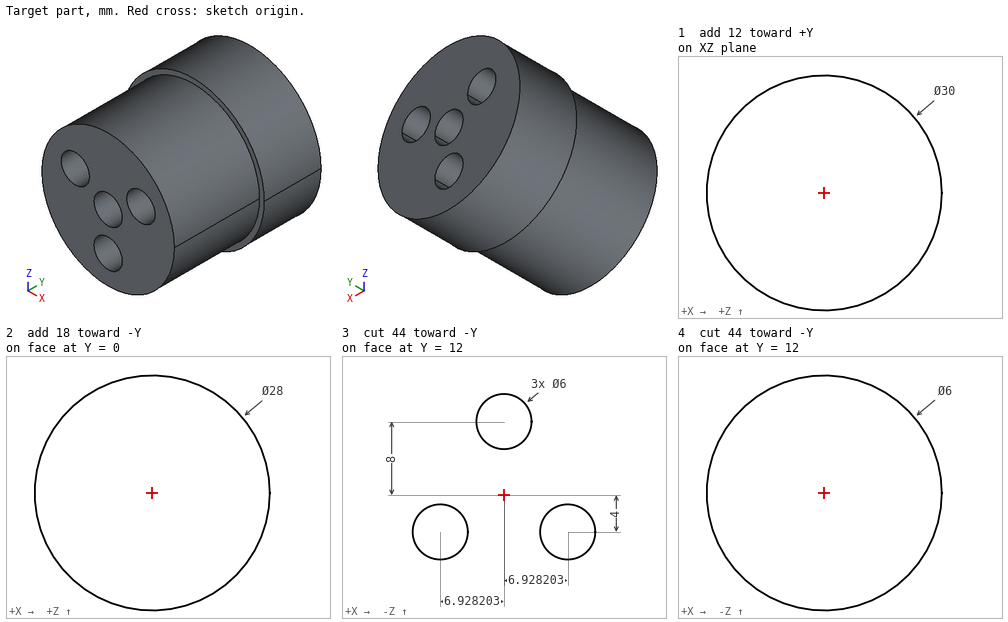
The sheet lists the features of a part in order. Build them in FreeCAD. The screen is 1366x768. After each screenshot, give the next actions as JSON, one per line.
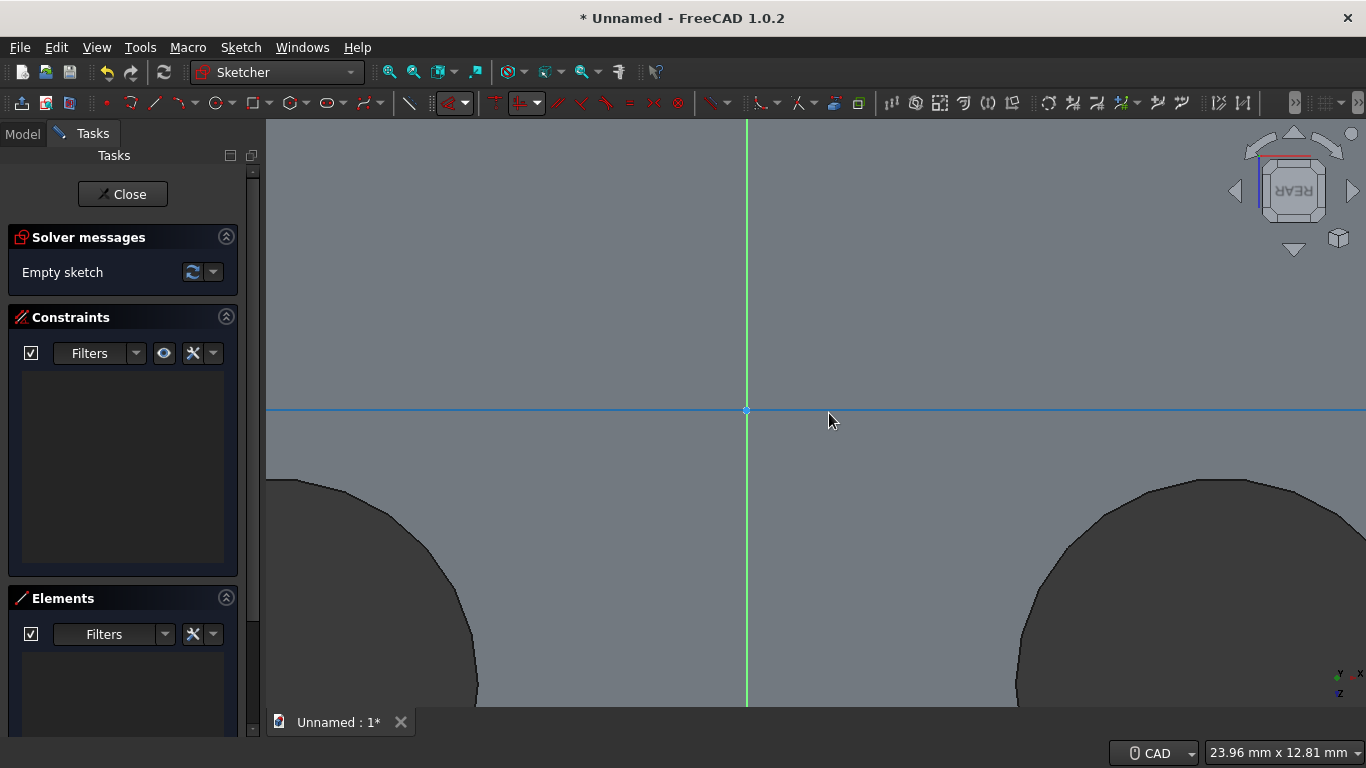
{"action": "left_click", "coordinate": [216, 104]}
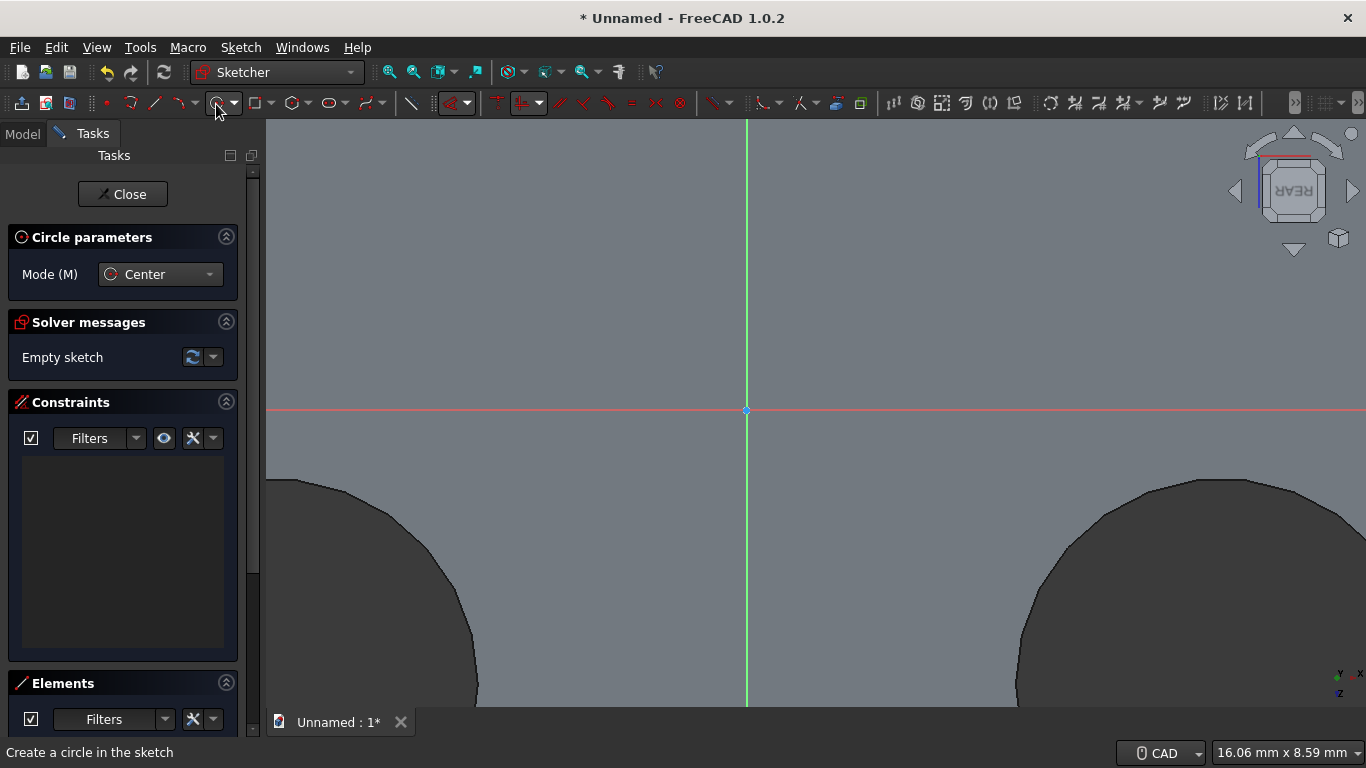
{"action": "left_click", "coordinate": [747, 410]}
{"action": "left_click", "coordinate": [892, 265]}
{"action": "key", "text": "Escape"}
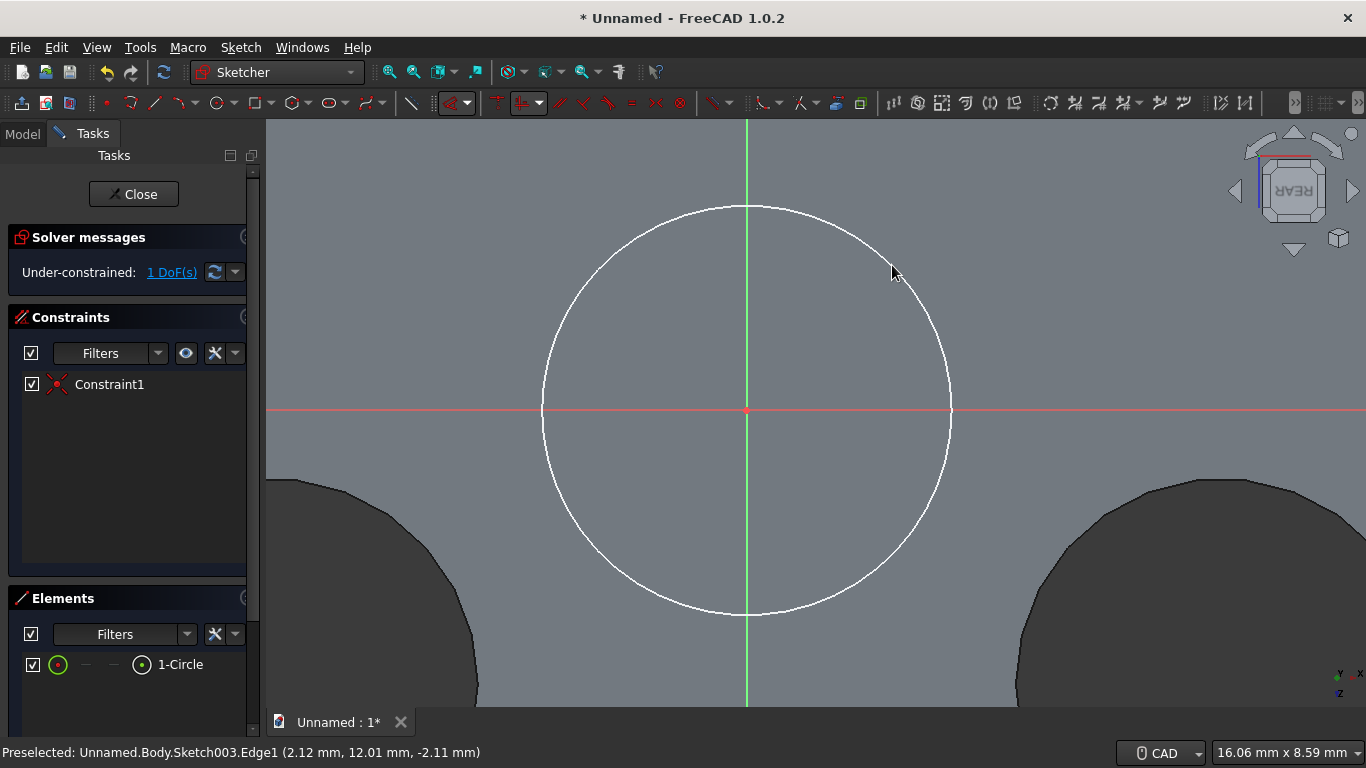
{"action": "left_click", "coordinate": [891, 265]}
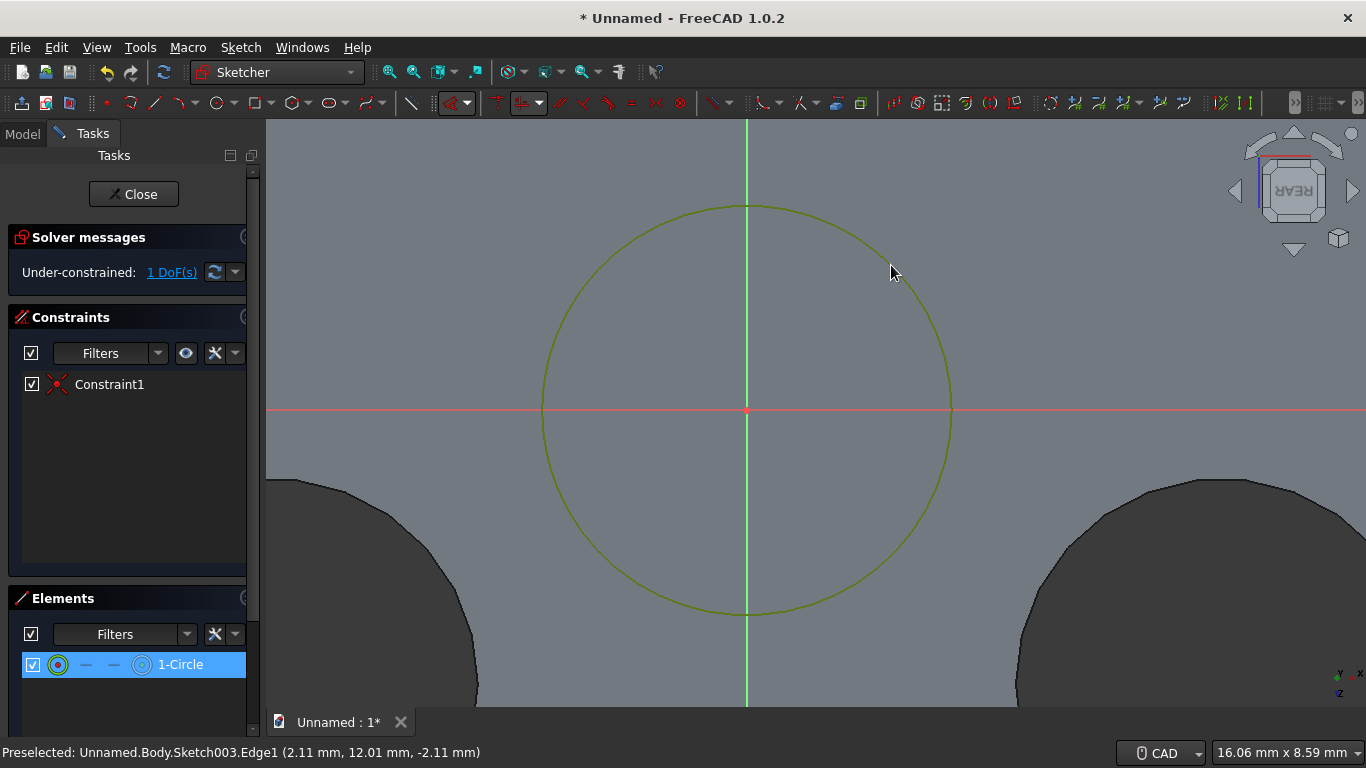
{"action": "left_click", "coordinate": [470, 104]}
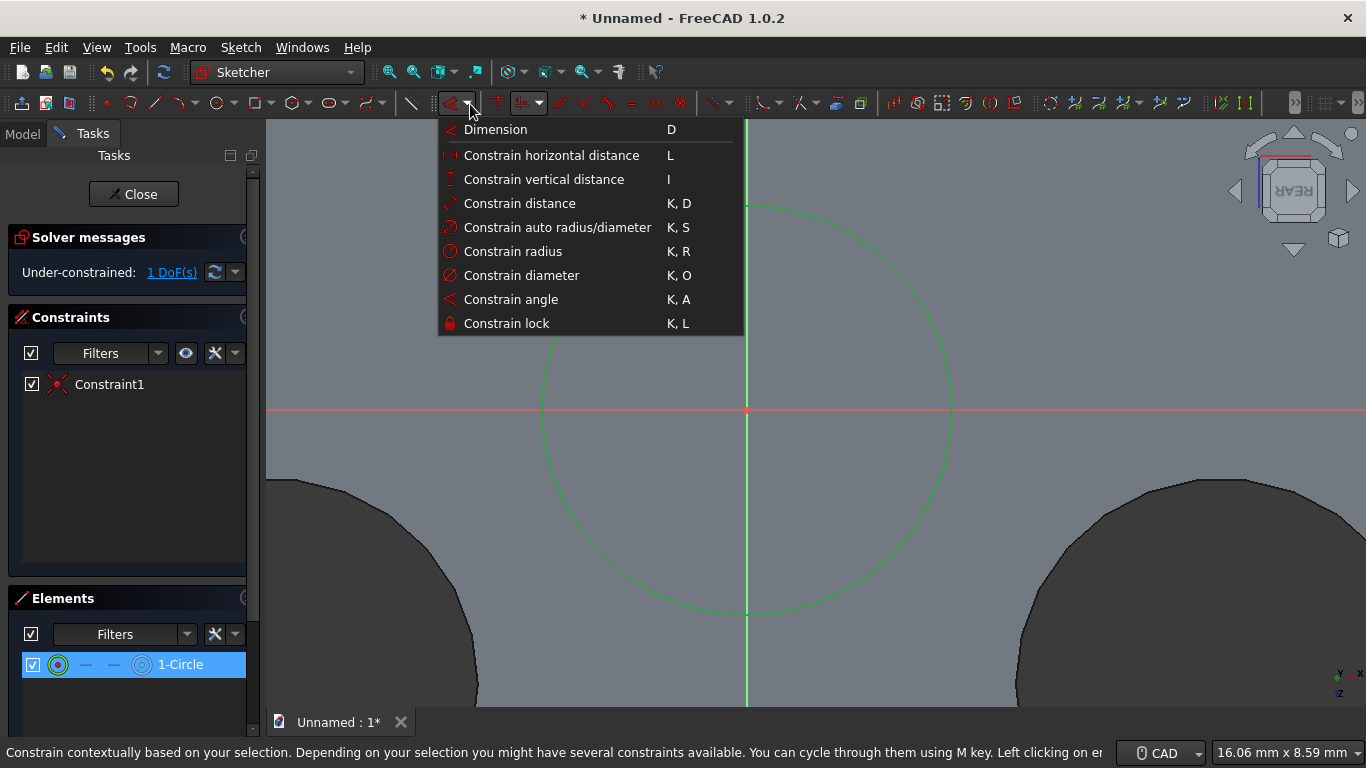
{"action": "left_click", "coordinate": [591, 275]}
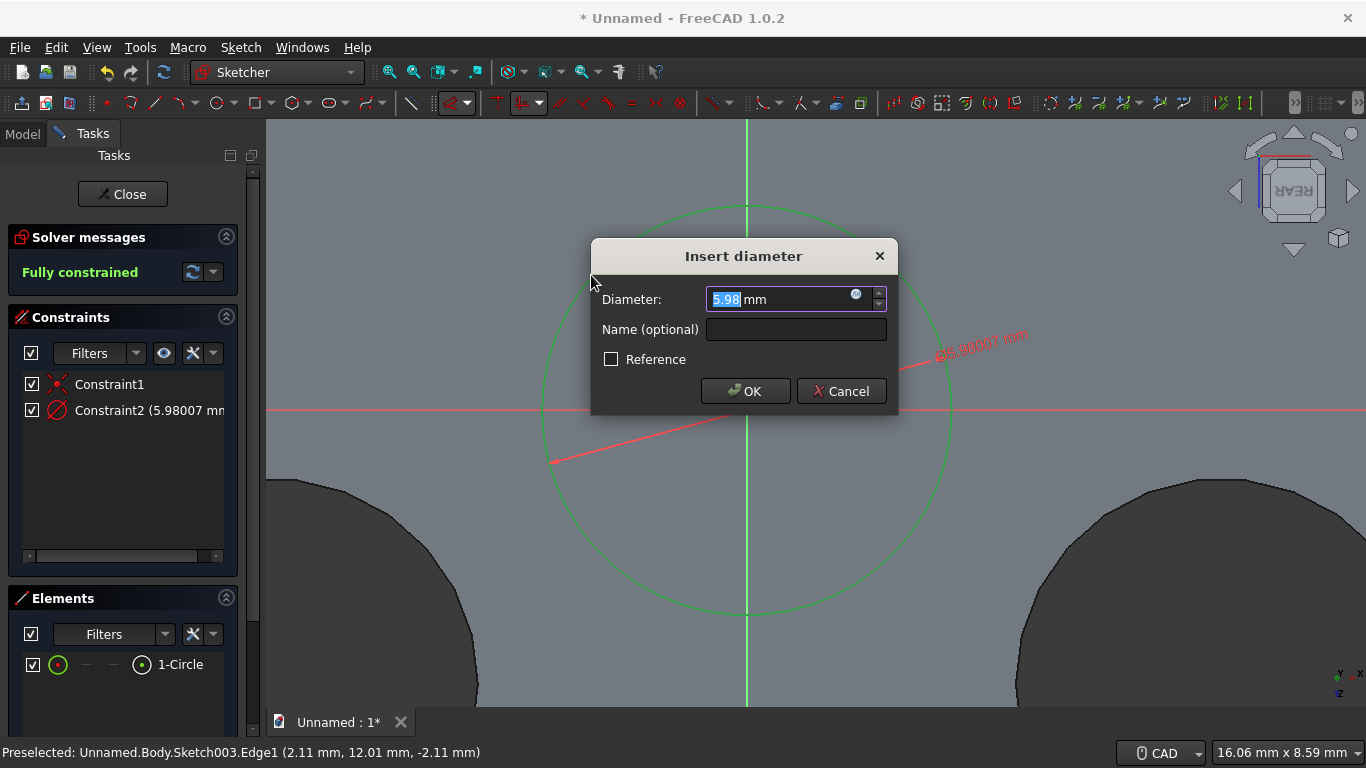
{"action": "type", "text": "6"}
{"action": "key", "text": "Return"}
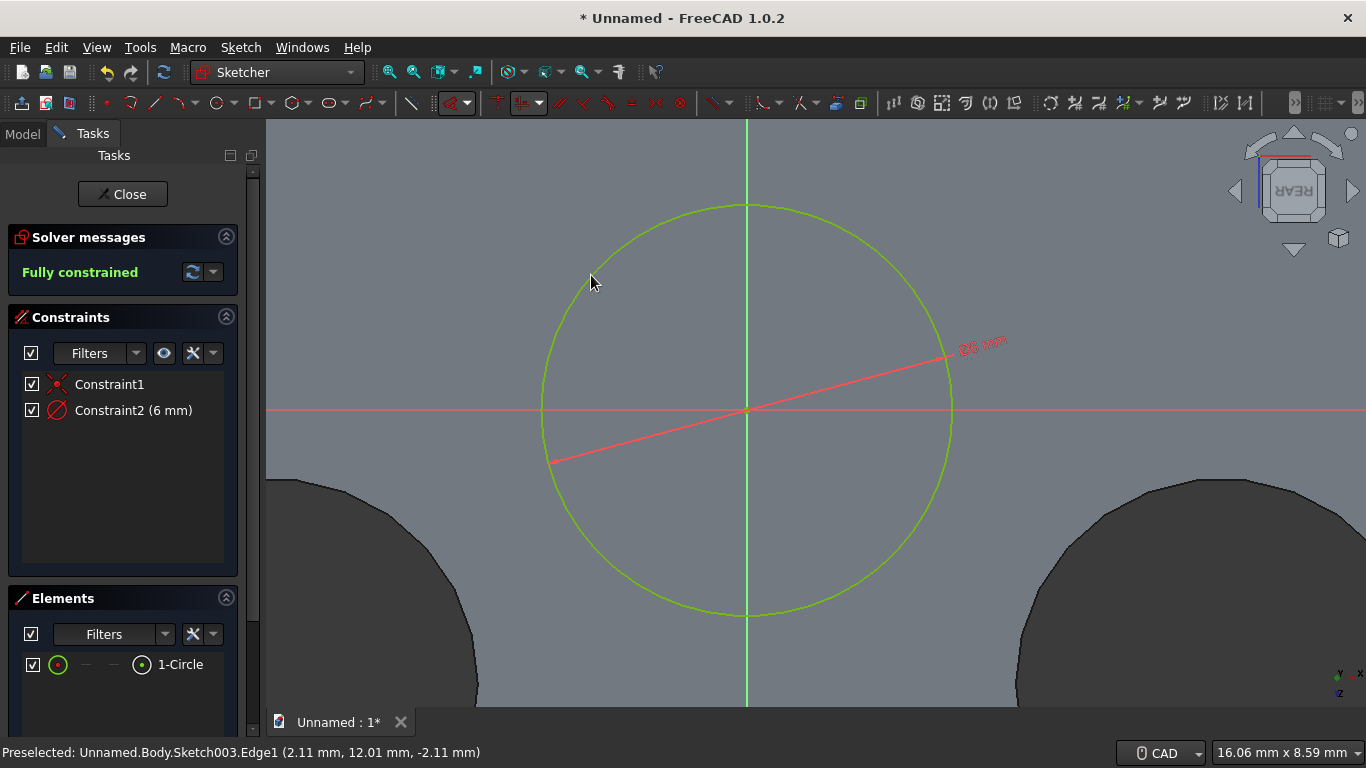
{"action": "left_click", "coordinate": [123, 194]}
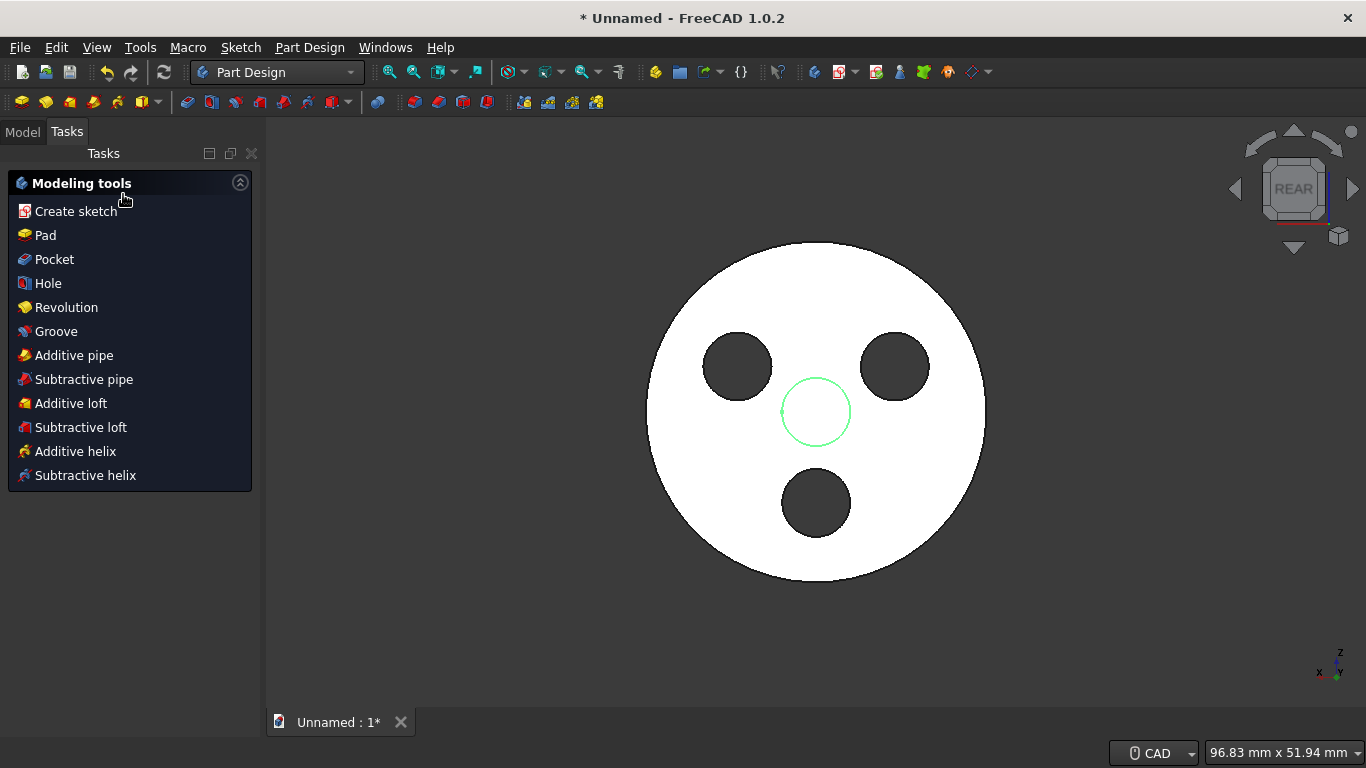
{"action": "left_click", "coordinate": [188, 102]}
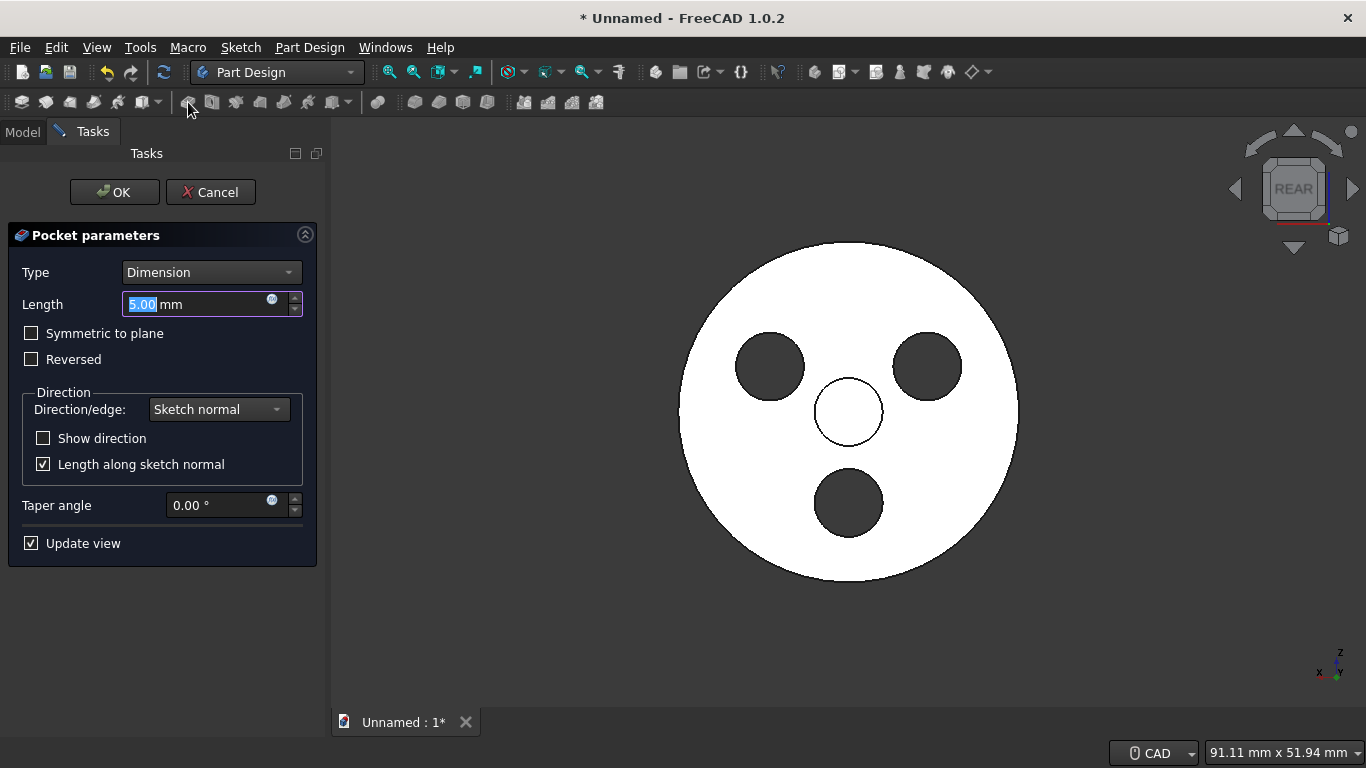
{"action": "type", "text": "44"}
{"action": "key", "text": "Tab"}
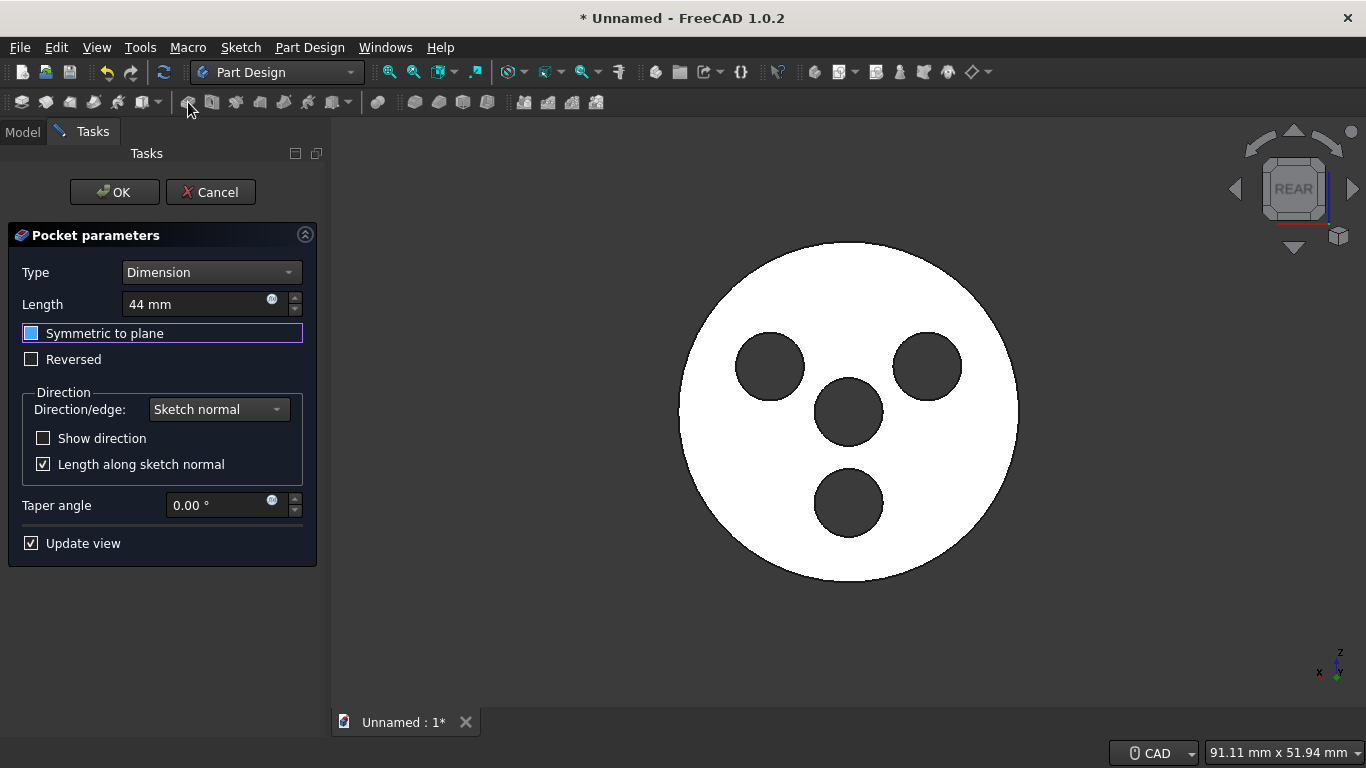
{"action": "left_click", "coordinate": [115, 192]}